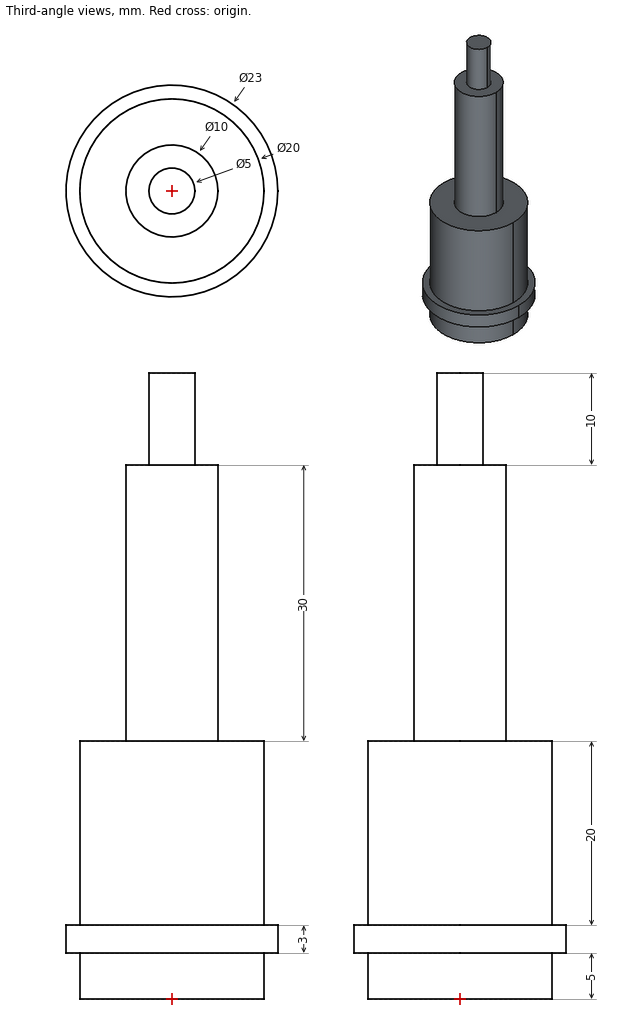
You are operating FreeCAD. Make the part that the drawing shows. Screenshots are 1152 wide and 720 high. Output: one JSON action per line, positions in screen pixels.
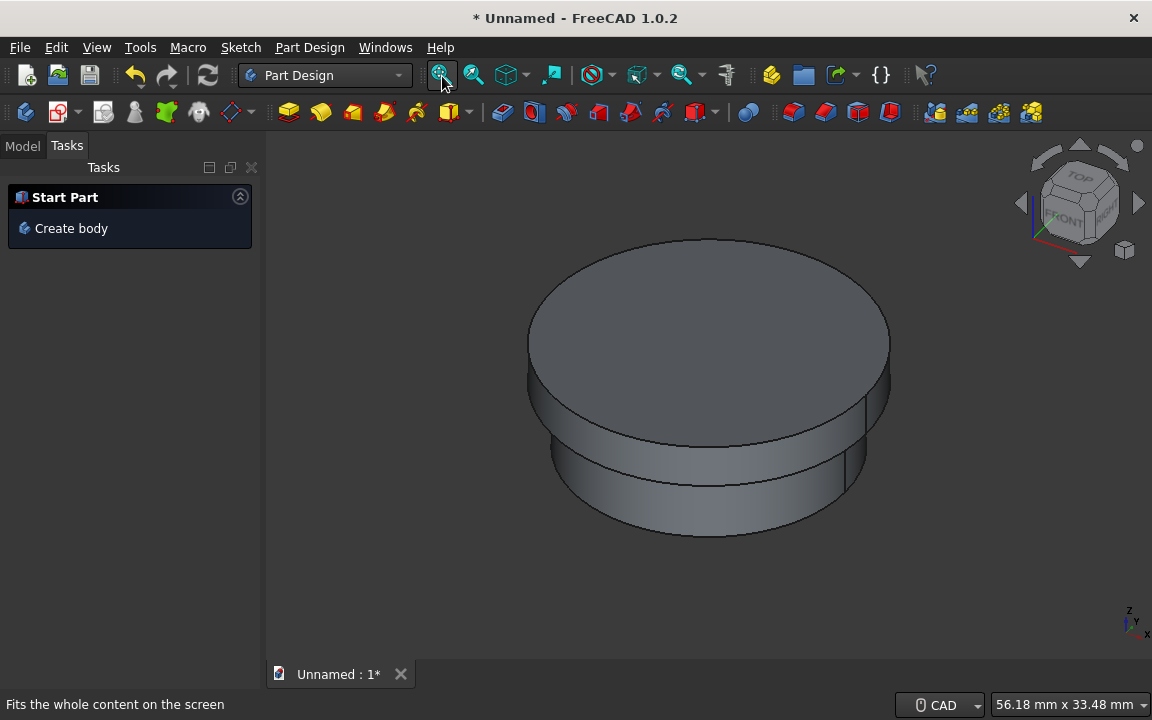
{"action": "left_click", "coordinate": [709, 342]}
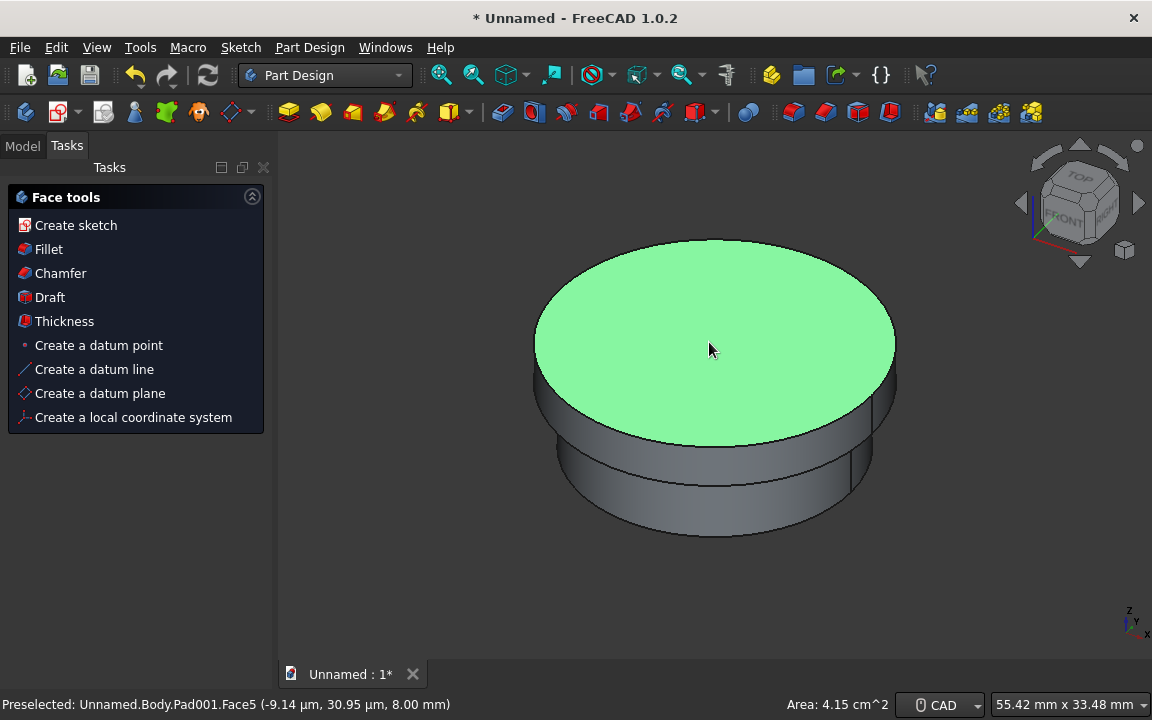
{"action": "left_click", "coordinate": [58, 112]}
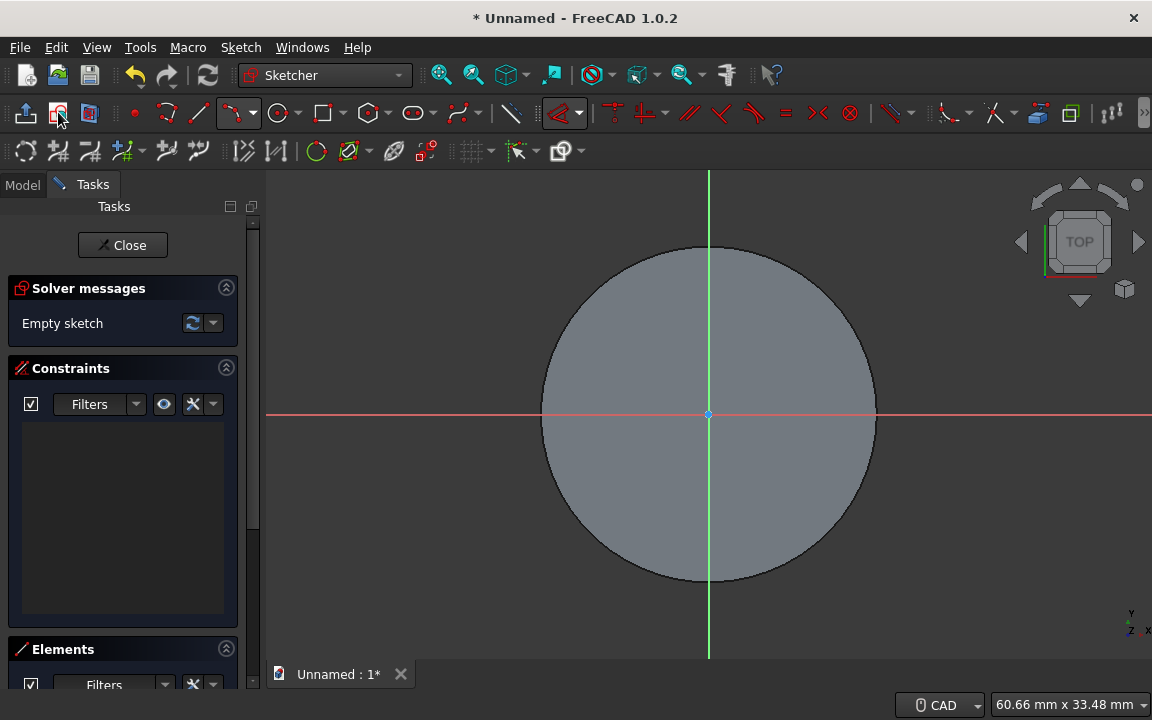
{"action": "left_click", "coordinate": [278, 114]}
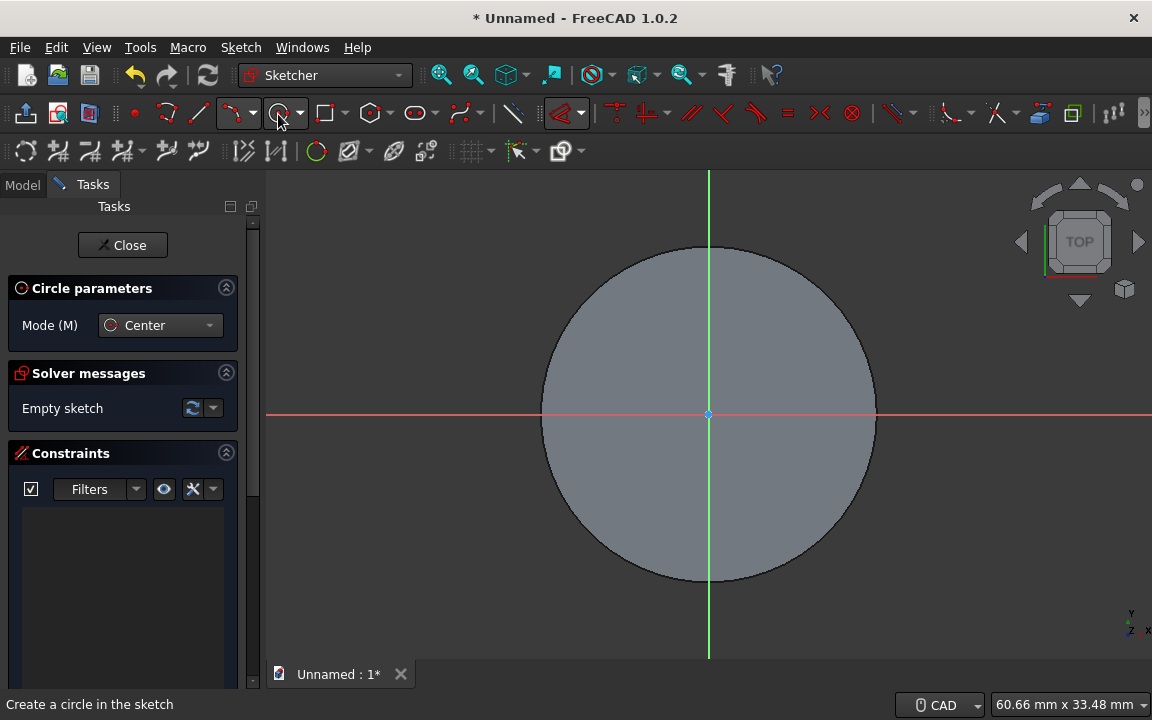
{"action": "left_click", "coordinate": [709, 414]}
{"action": "mouse_move", "coordinate": [812, 311]}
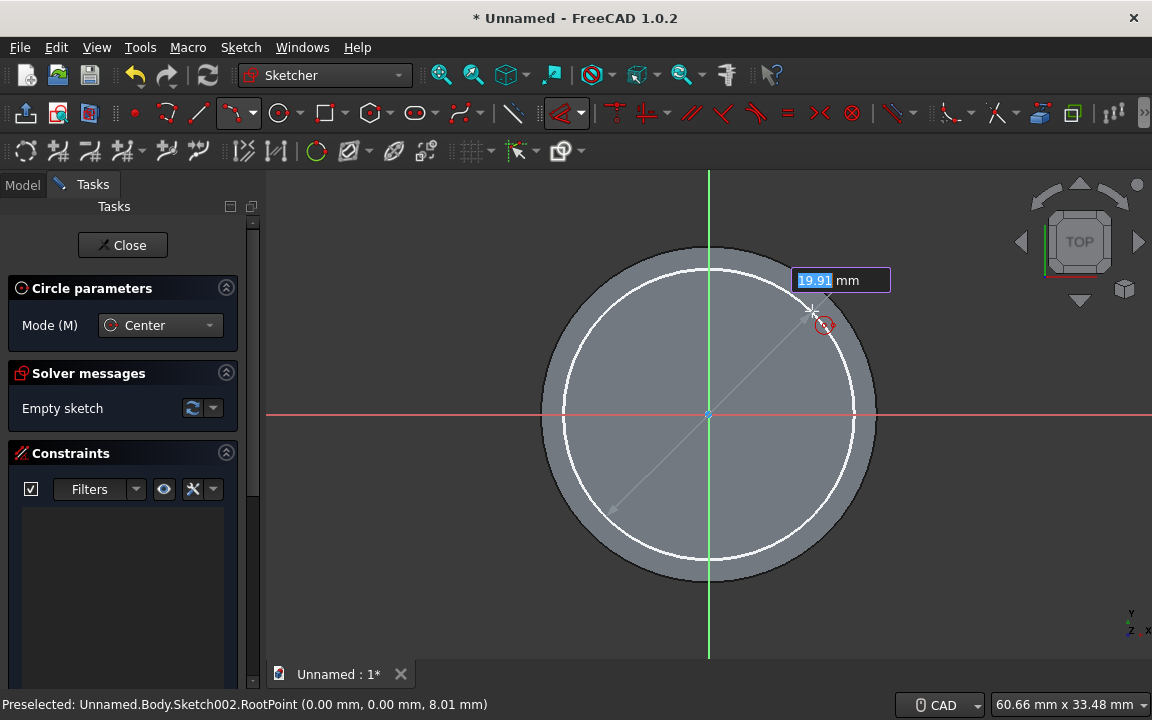
{"action": "type", "text": "20"}
{"action": "key", "text": "Return"}
{"action": "key", "text": "Escape"}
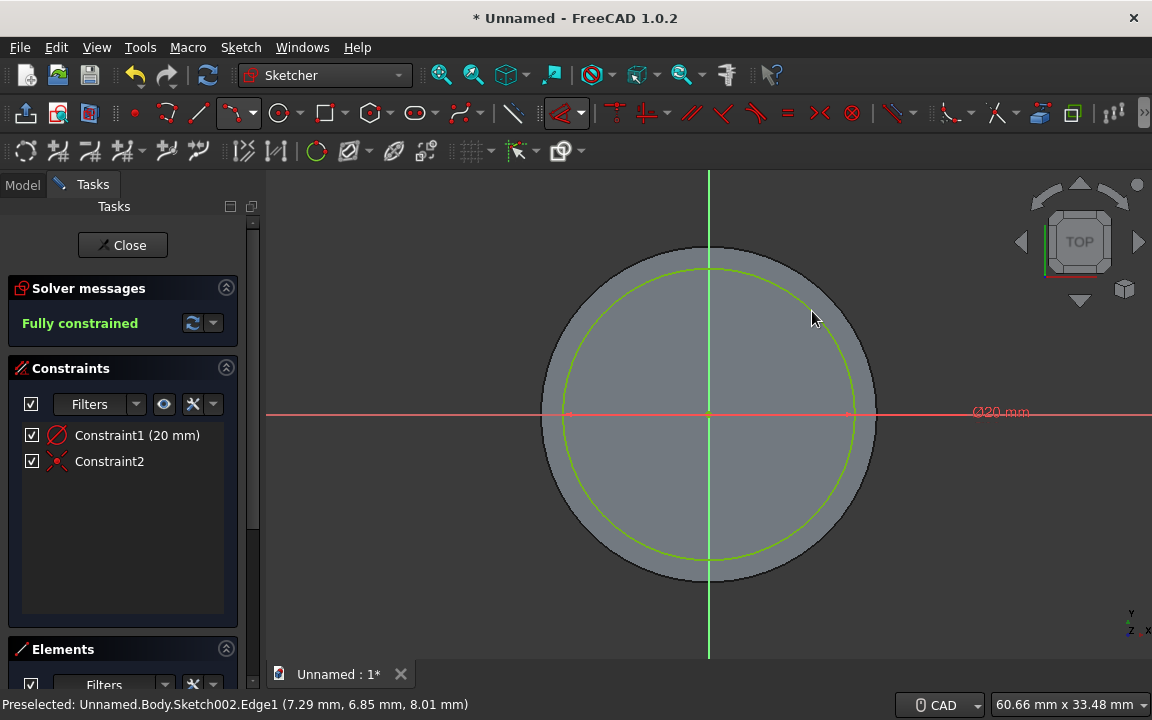
{"action": "left_click", "coordinate": [123, 245]}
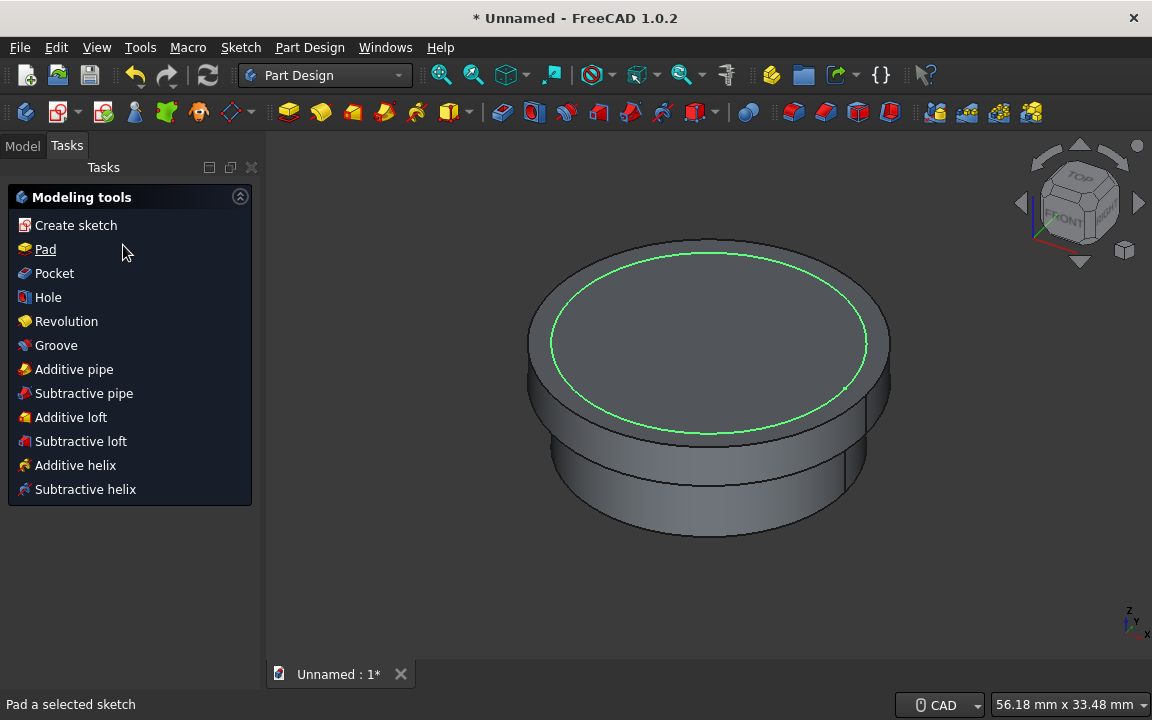
{"action": "left_click", "coordinate": [290, 112]}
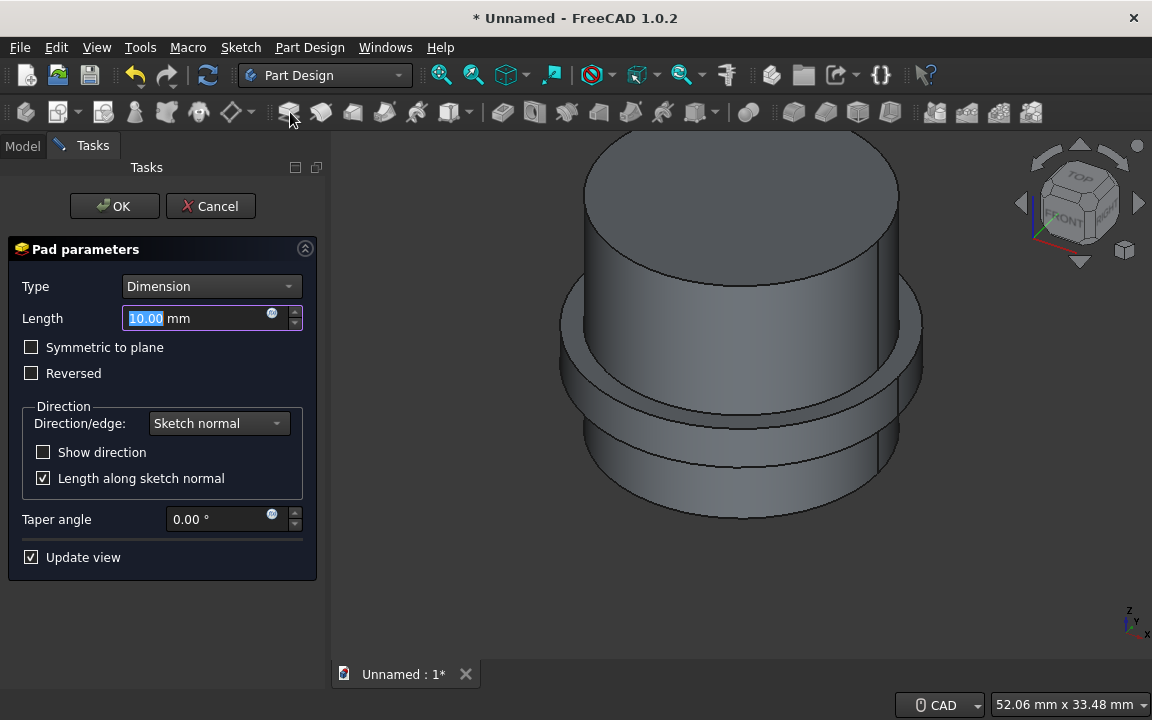
{"action": "type", "text": "20"}
{"action": "key", "text": "Tab"}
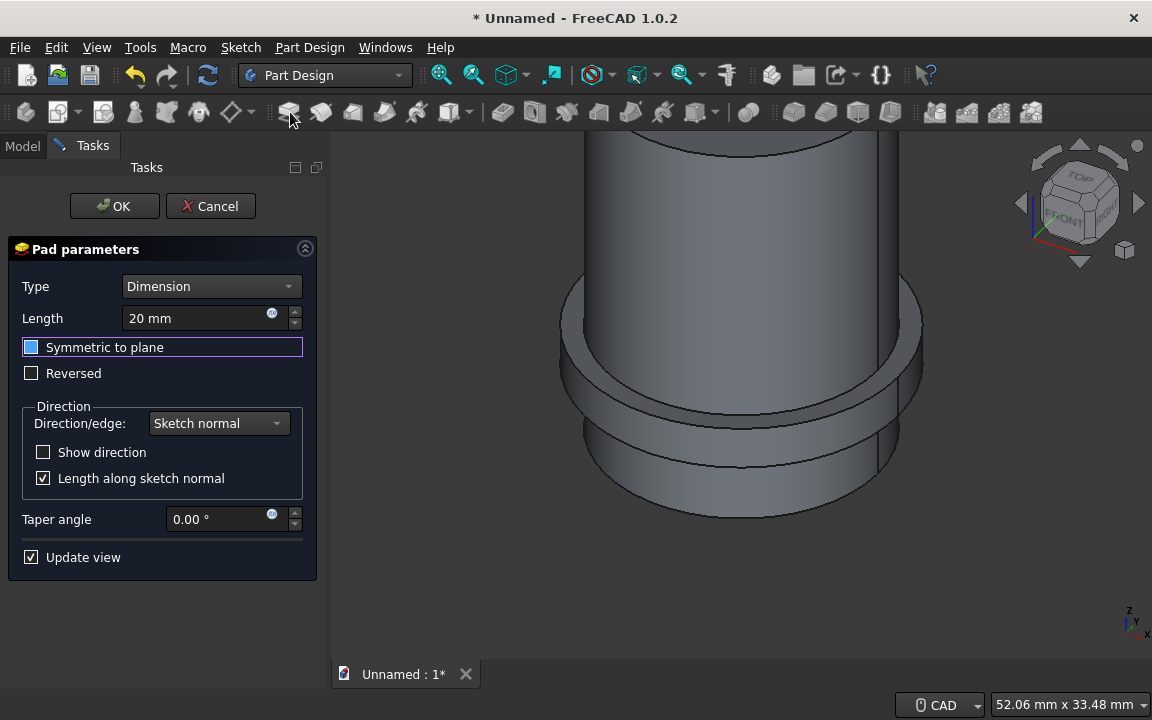
{"action": "left_click", "coordinate": [115, 206]}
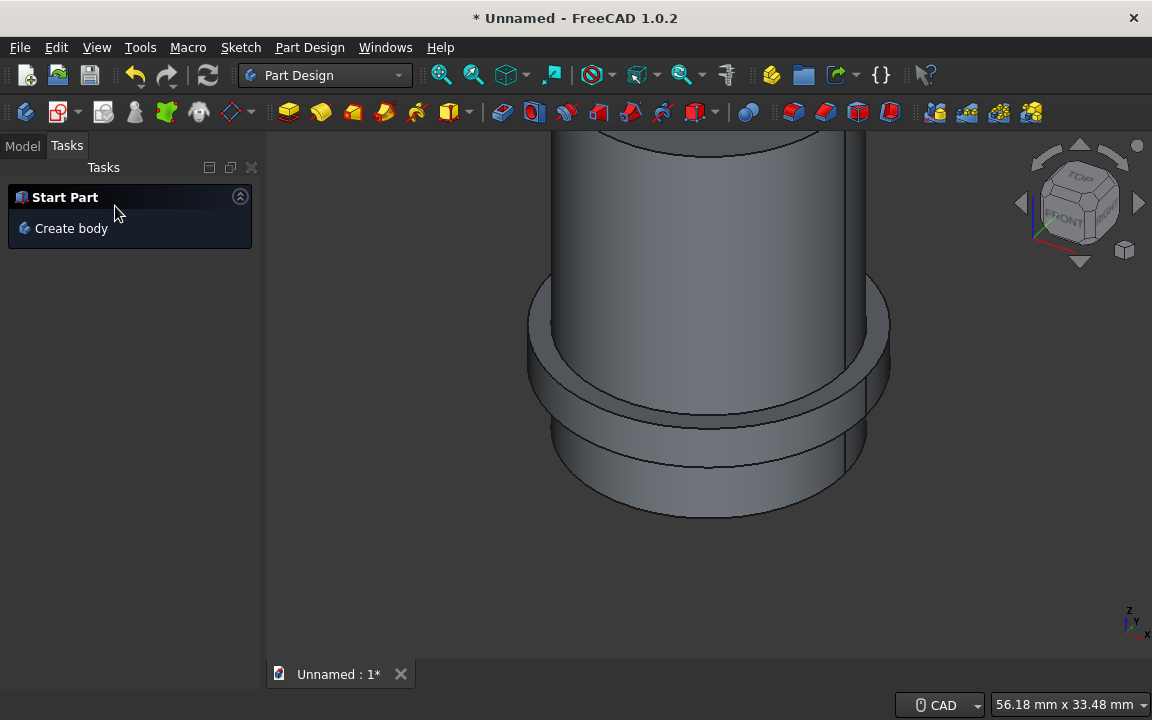
{"action": "left_click", "coordinate": [442, 76]}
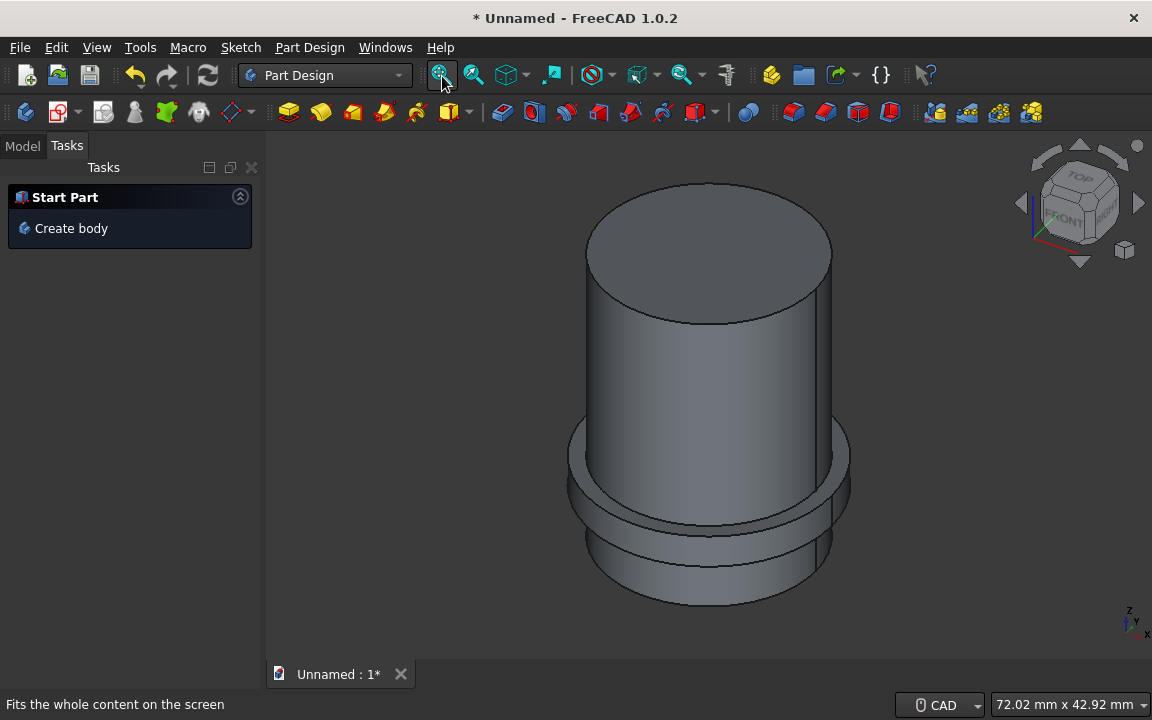
{"action": "left_click", "coordinate": [709, 253]}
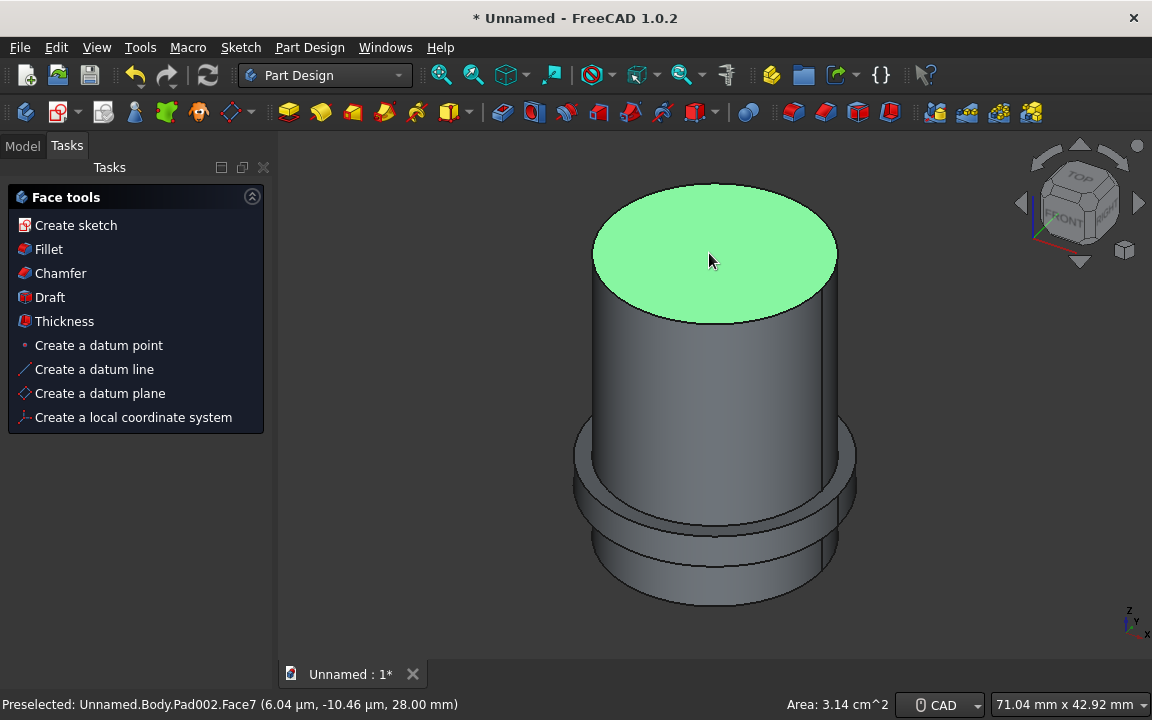
{"action": "left_click", "coordinate": [58, 112]}